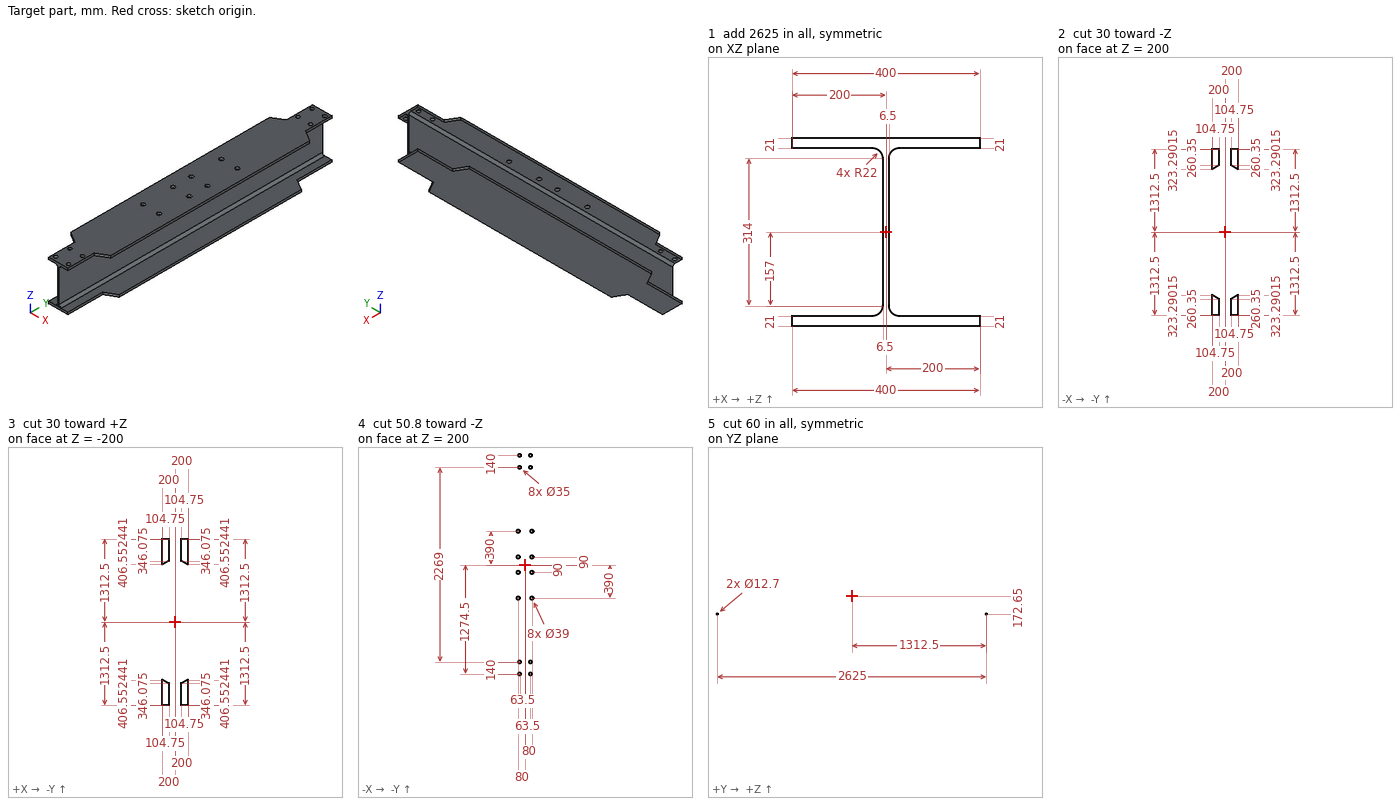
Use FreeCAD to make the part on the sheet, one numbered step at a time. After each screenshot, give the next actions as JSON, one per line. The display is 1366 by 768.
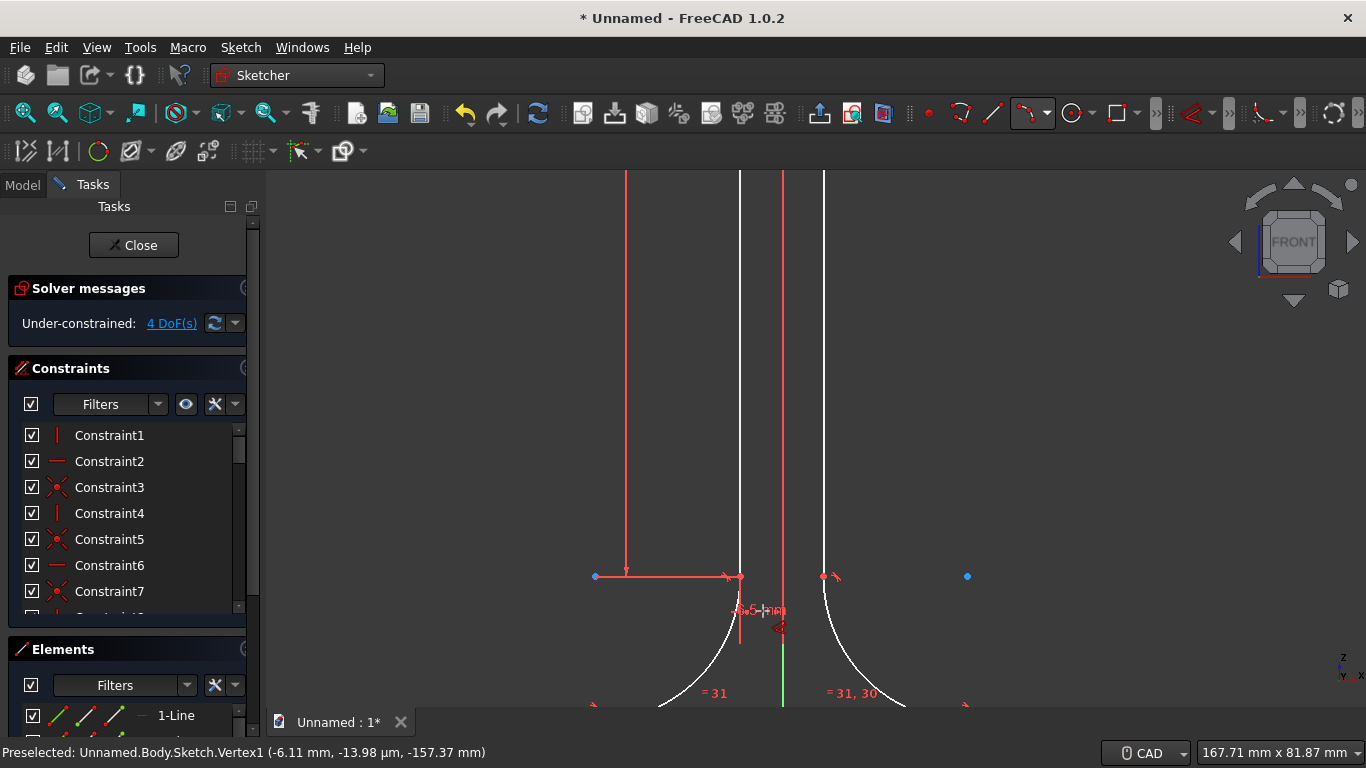
{"action": "scroll", "coordinate": [742, 578], "scroll_direction": "down", "scroll_amount": 10}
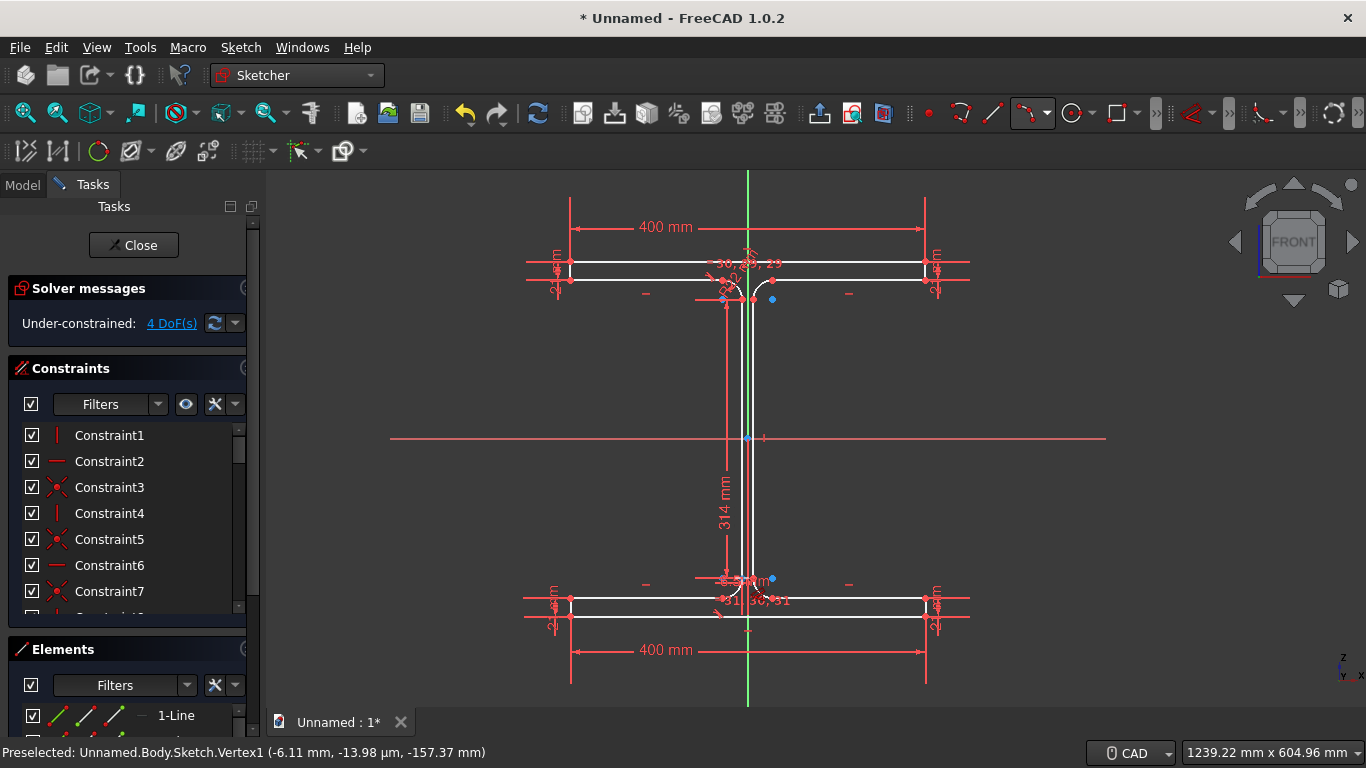
{"action": "left_click", "coordinate": [742, 578]}
{"action": "left_click", "coordinate": [708, 477]}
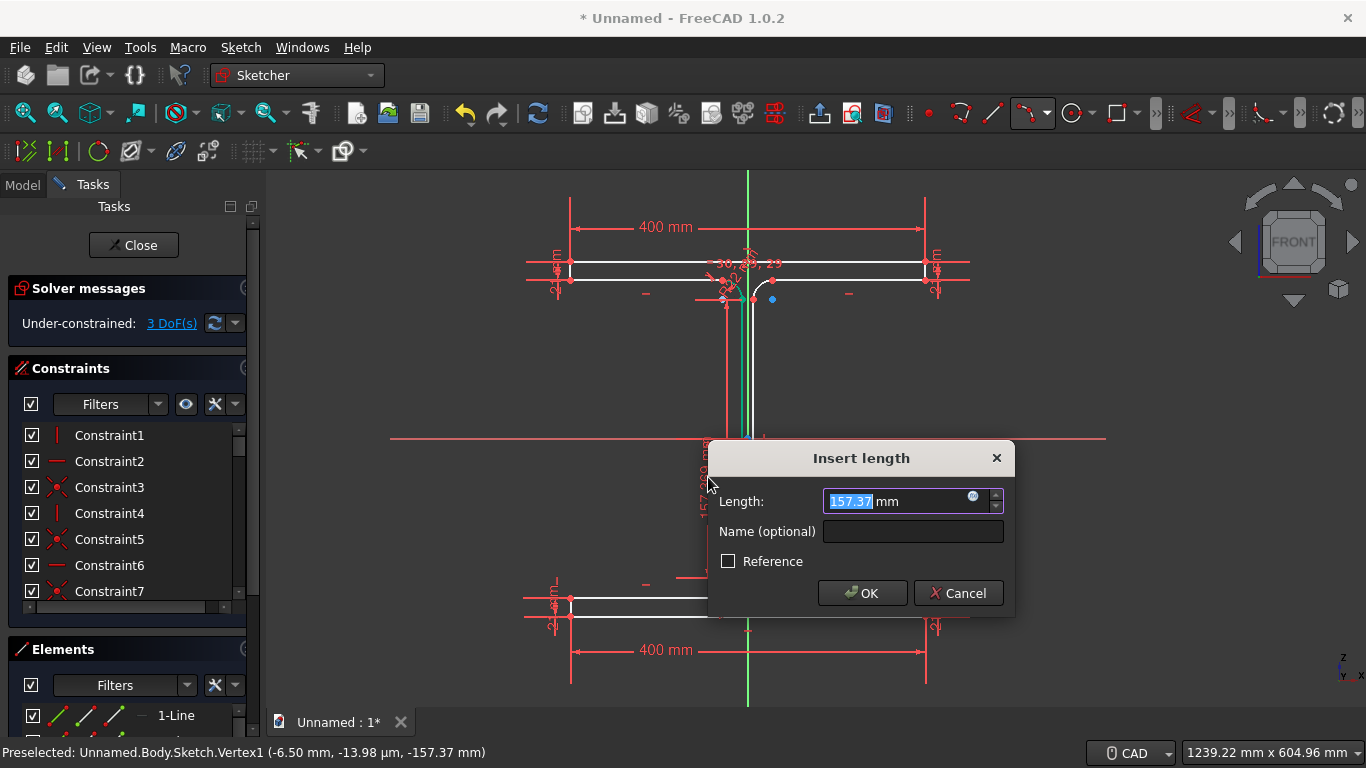
{"action": "type", "text": "157"}
{"action": "key", "text": "Return"}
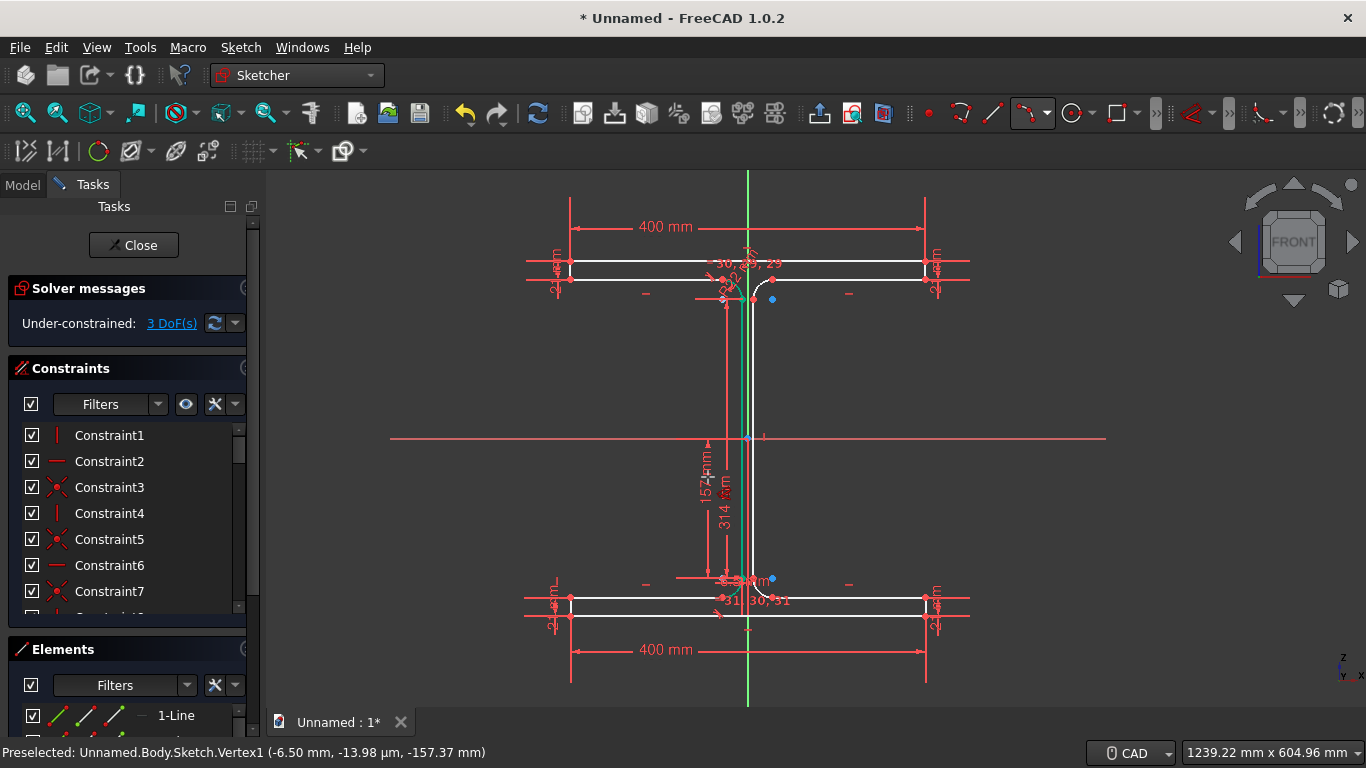
{"action": "left_click", "coordinate": [570, 280]}
{"action": "left_click", "coordinate": [618, 473]}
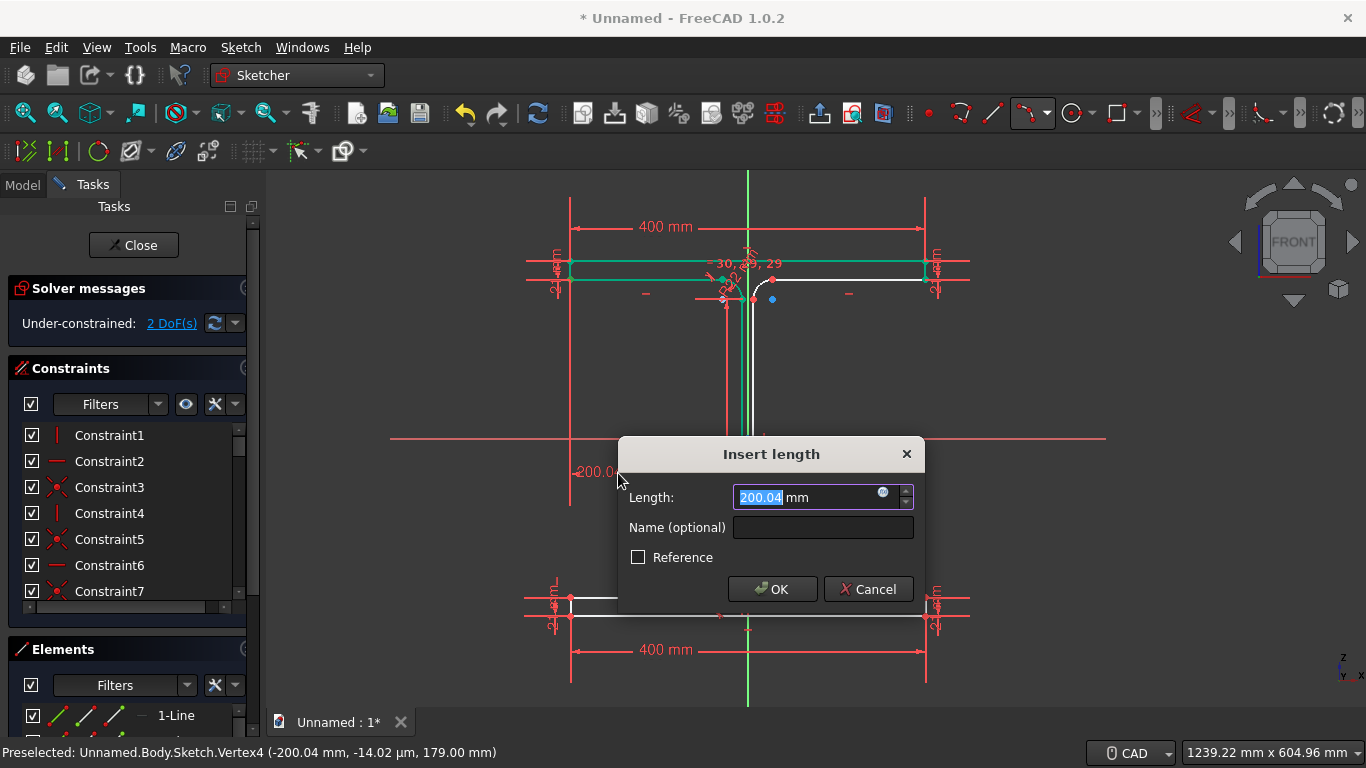
{"action": "type", "text": "200"}
{"action": "key", "text": "Return"}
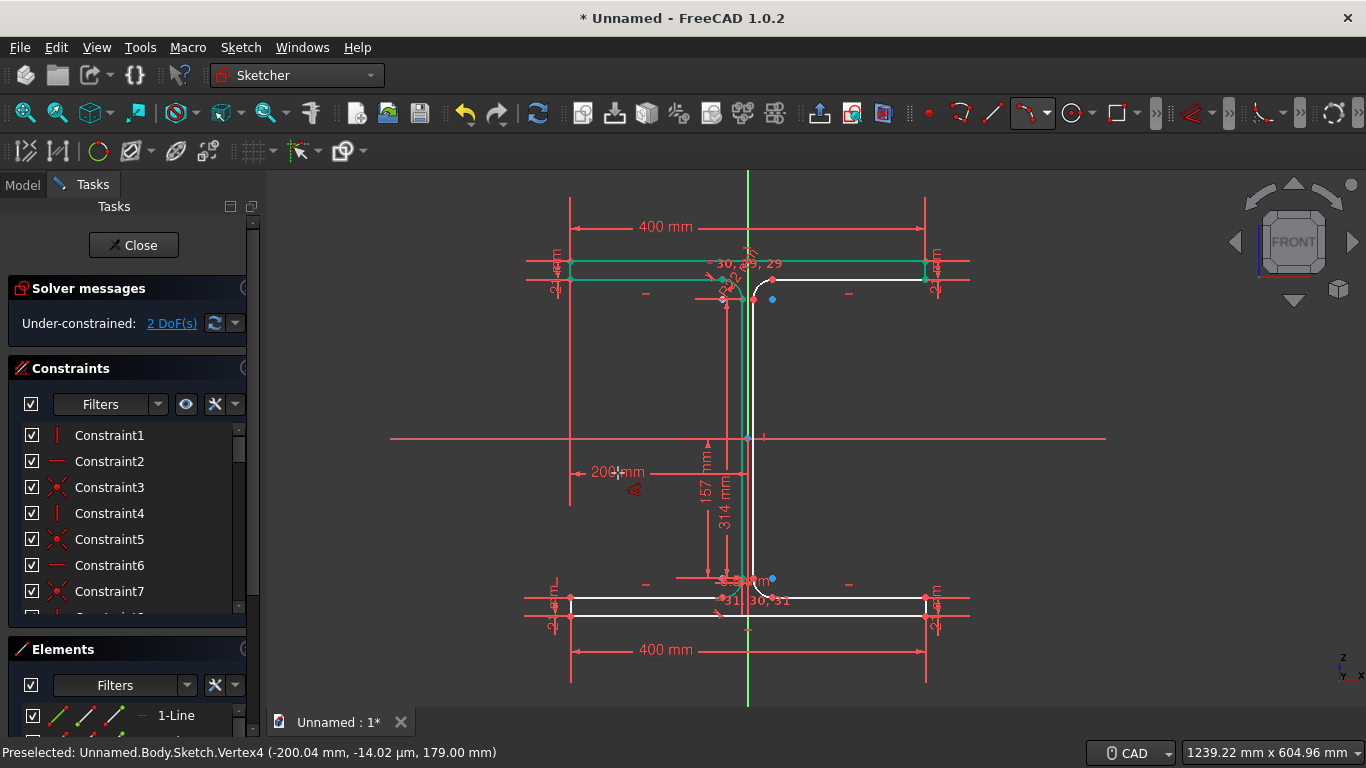
{"action": "scroll", "coordinate": [753, 299], "scroll_direction": "up", "scroll_amount": 10}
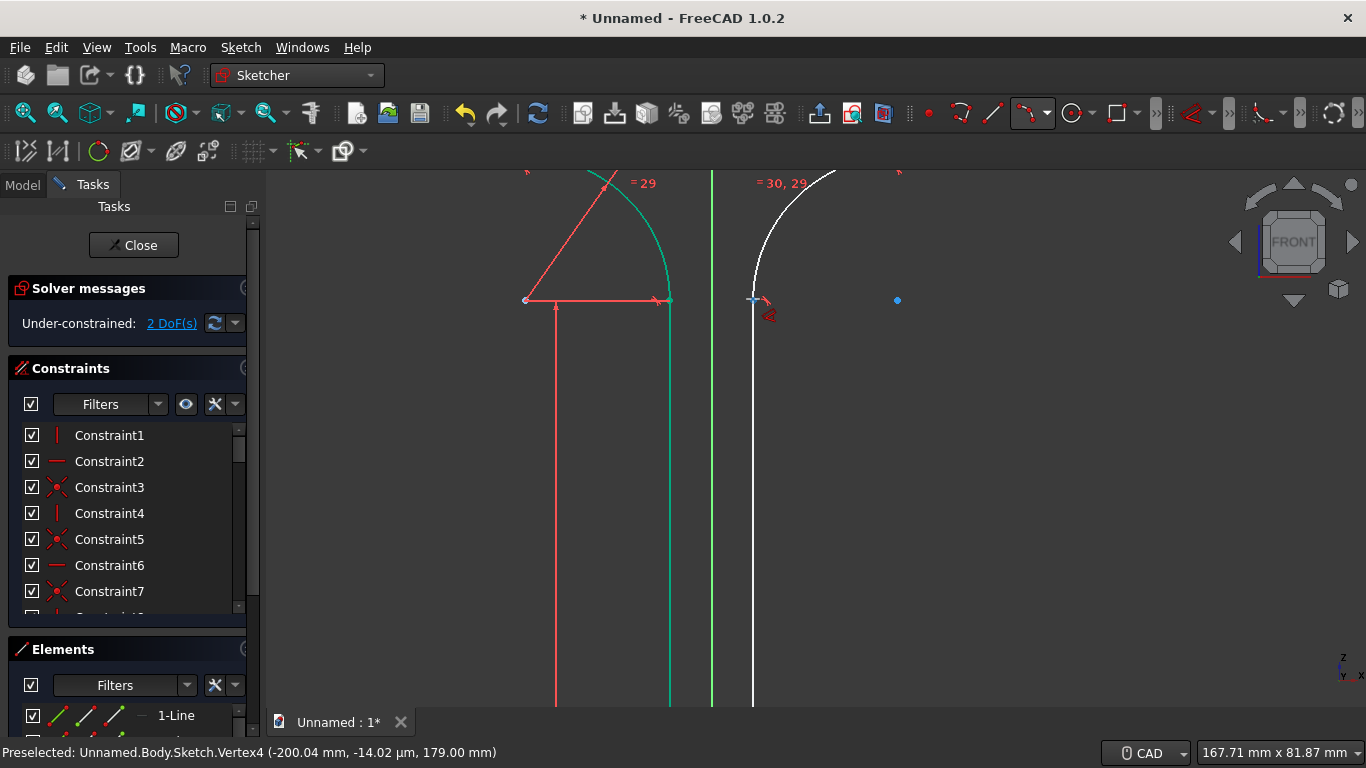
{"action": "left_click", "coordinate": [753, 301]}
{"action": "left_click", "coordinate": [733, 267]}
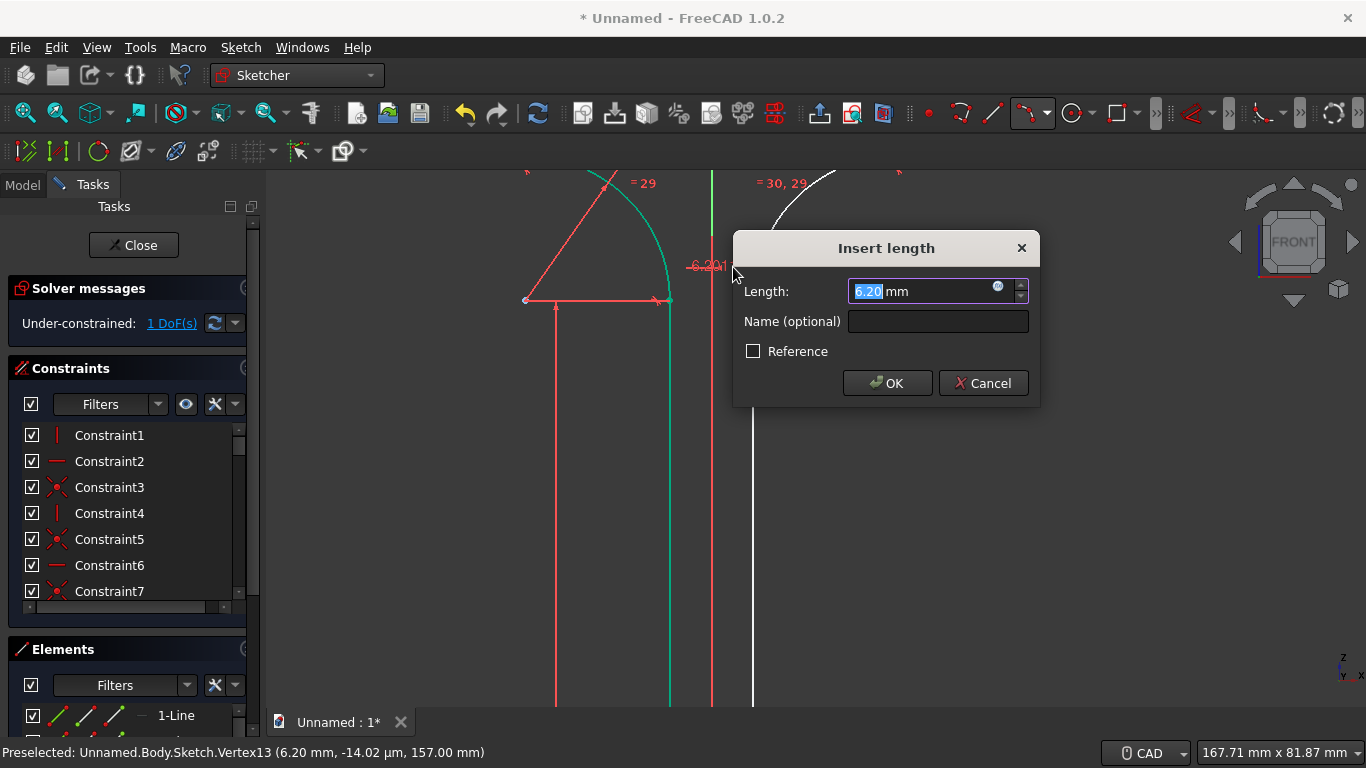
{"action": "type", "text": "6.5"}
{"action": "key", "text": "Return"}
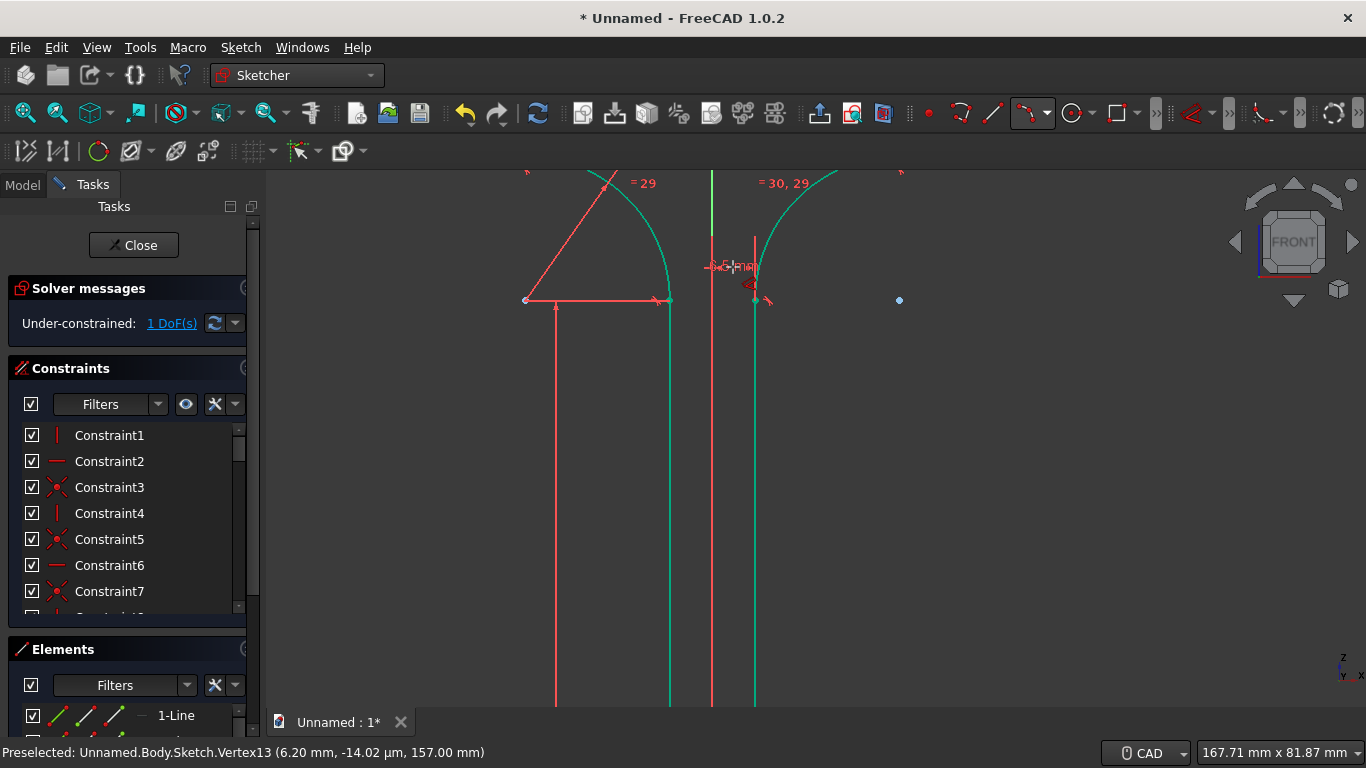
{"action": "scroll", "coordinate": [753, 299], "scroll_direction": "down", "scroll_amount": 10}